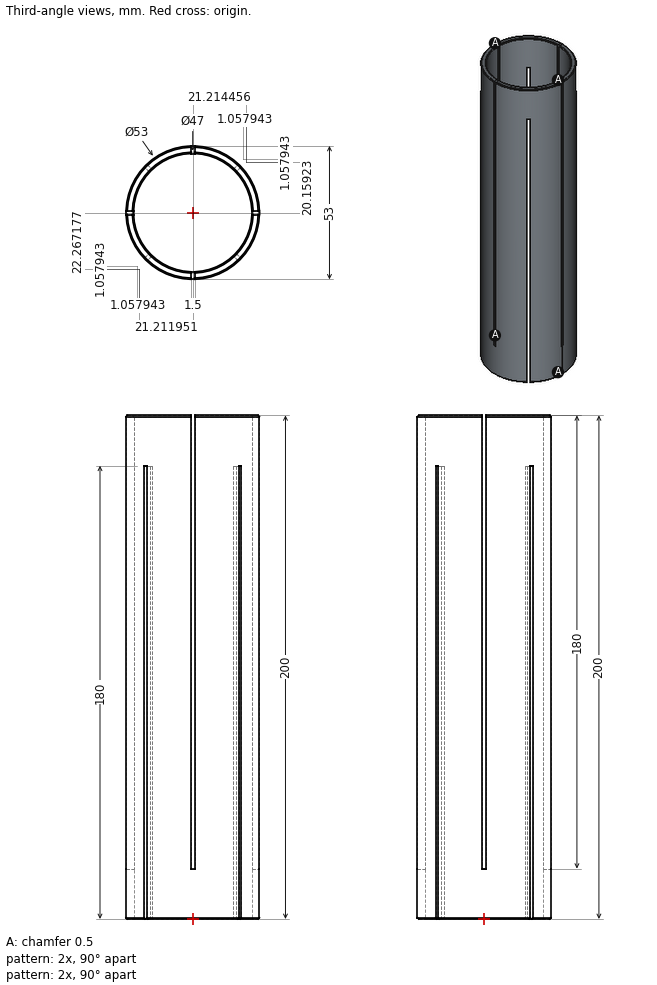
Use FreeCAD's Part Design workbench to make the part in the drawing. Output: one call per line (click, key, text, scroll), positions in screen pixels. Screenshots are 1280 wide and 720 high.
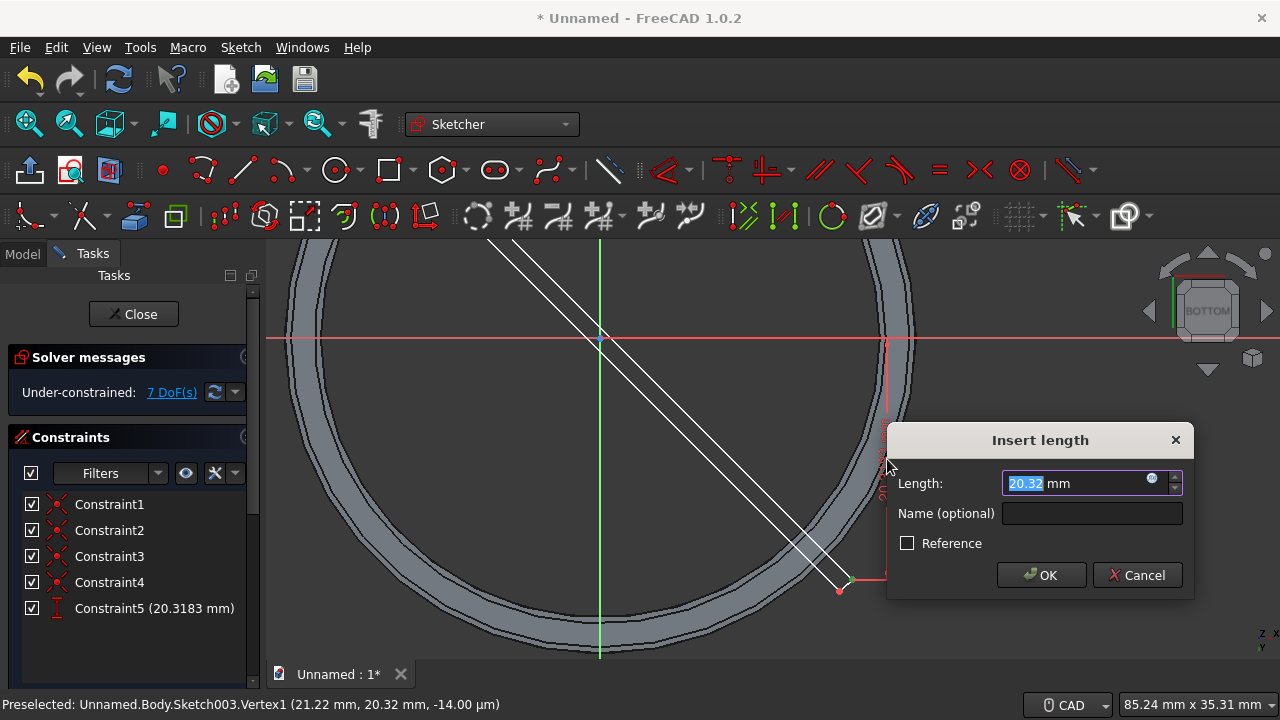
text(20.15923)
key(Return)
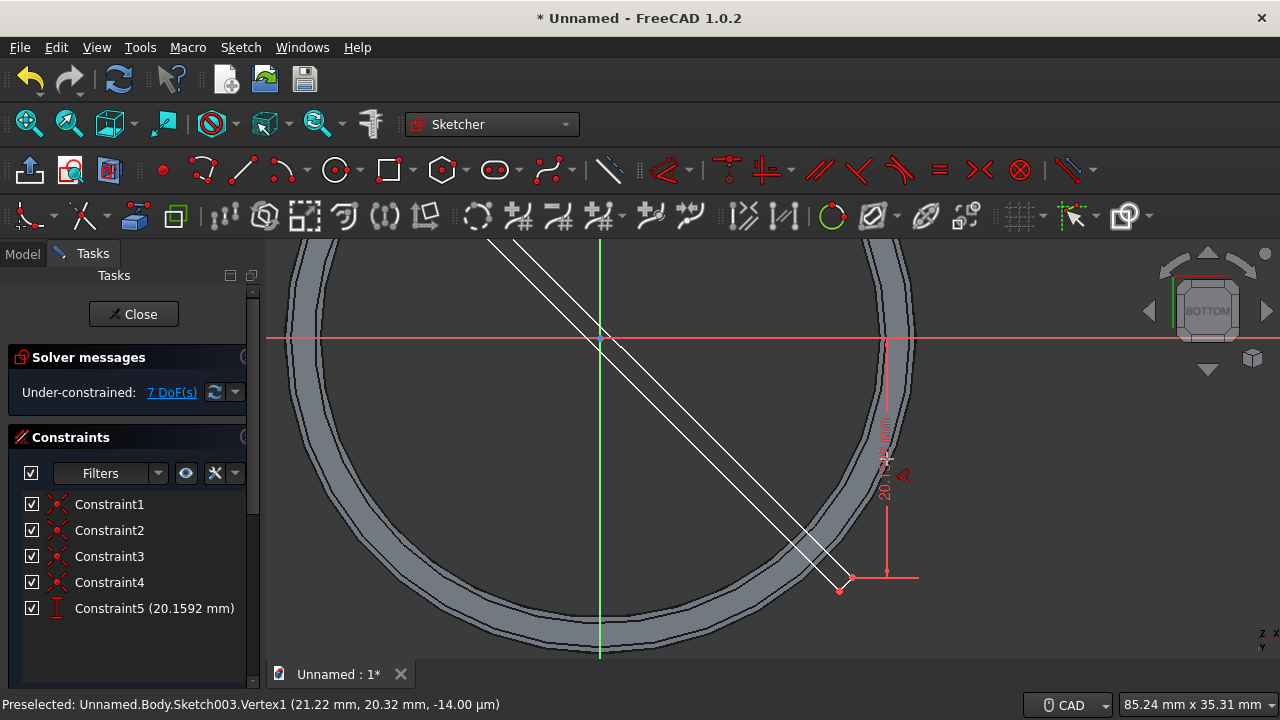
scroll(839, 592, down, 3)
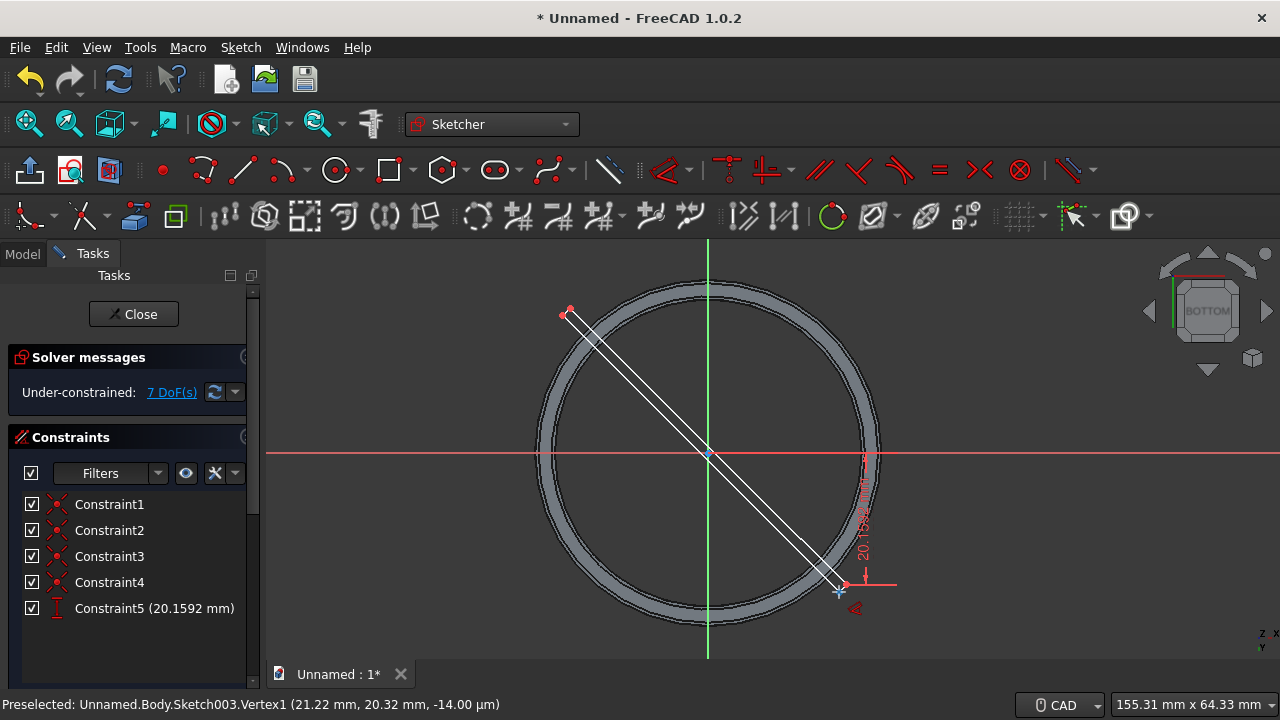
scroll(566, 312, up, 9)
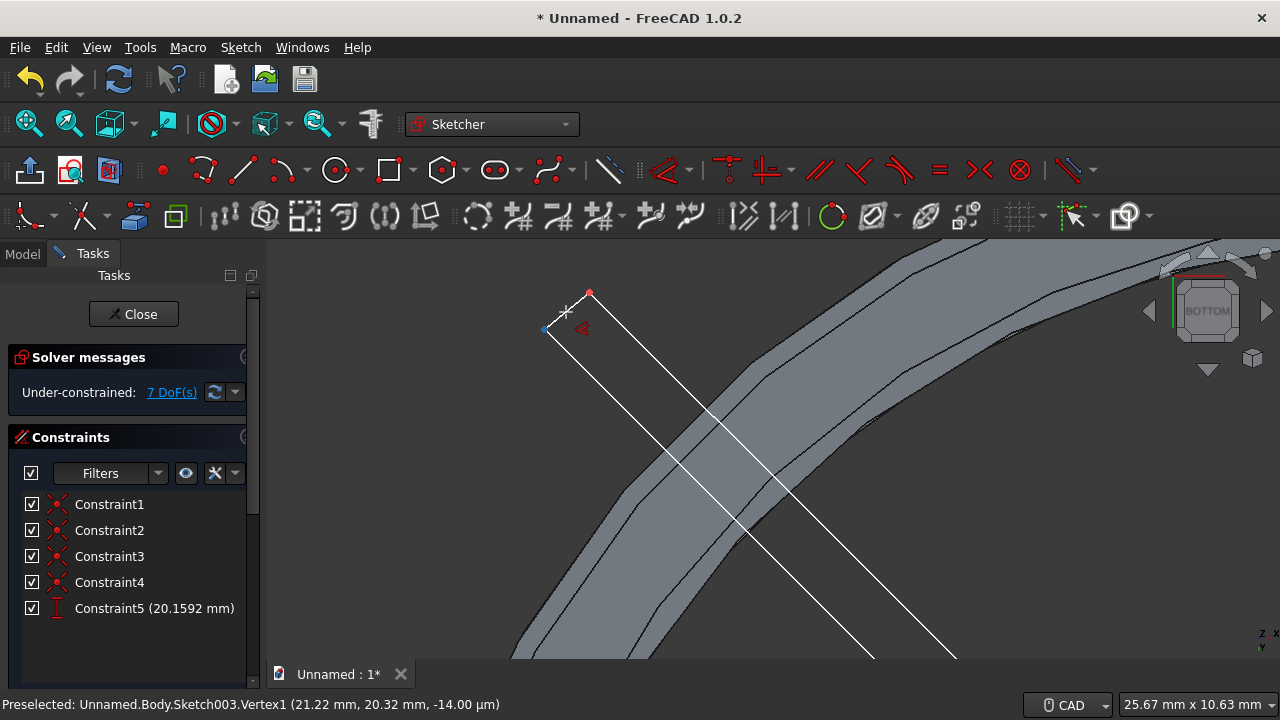
click(567, 311)
click(557, 363)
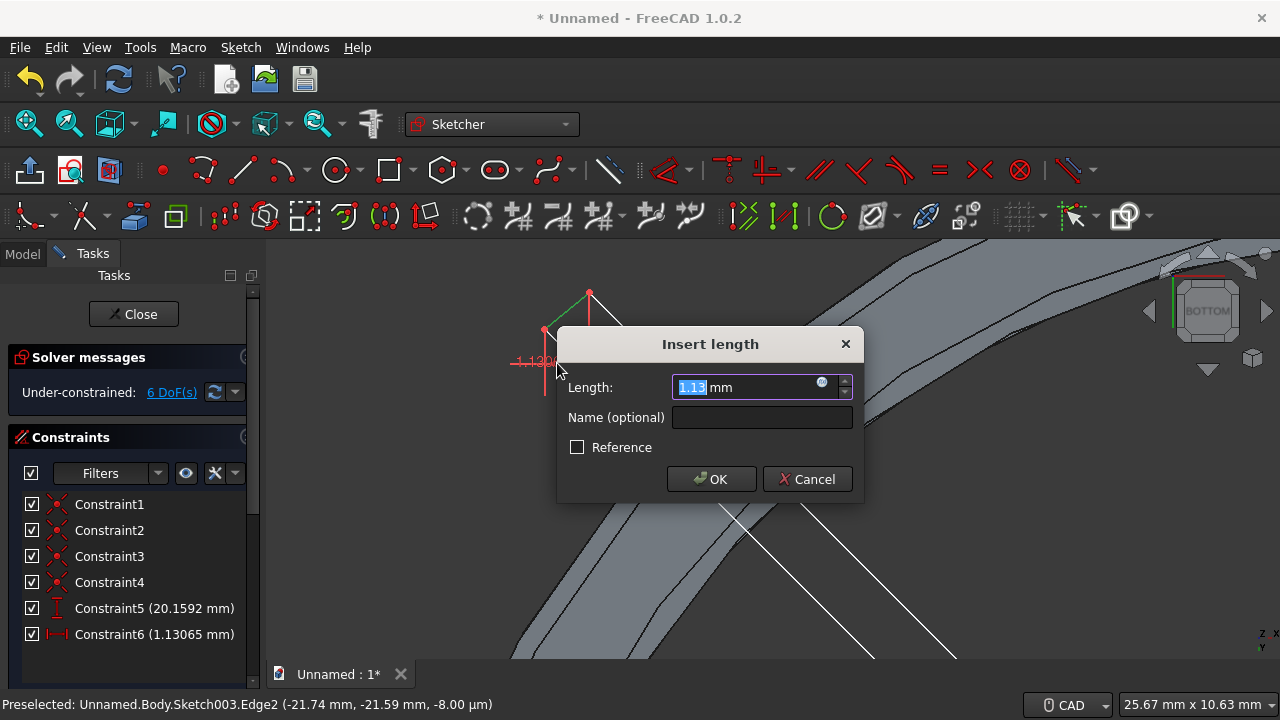
text(1.057943)
key(Return)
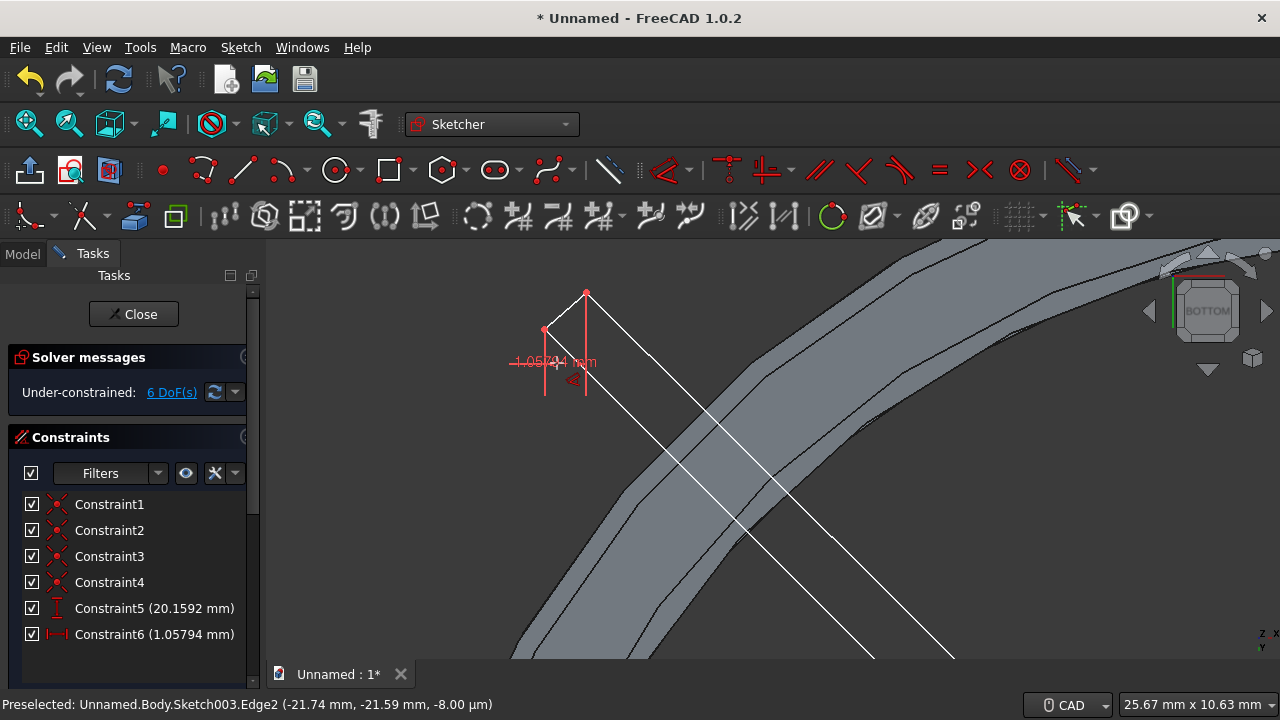
click(574, 304)
click(511, 311)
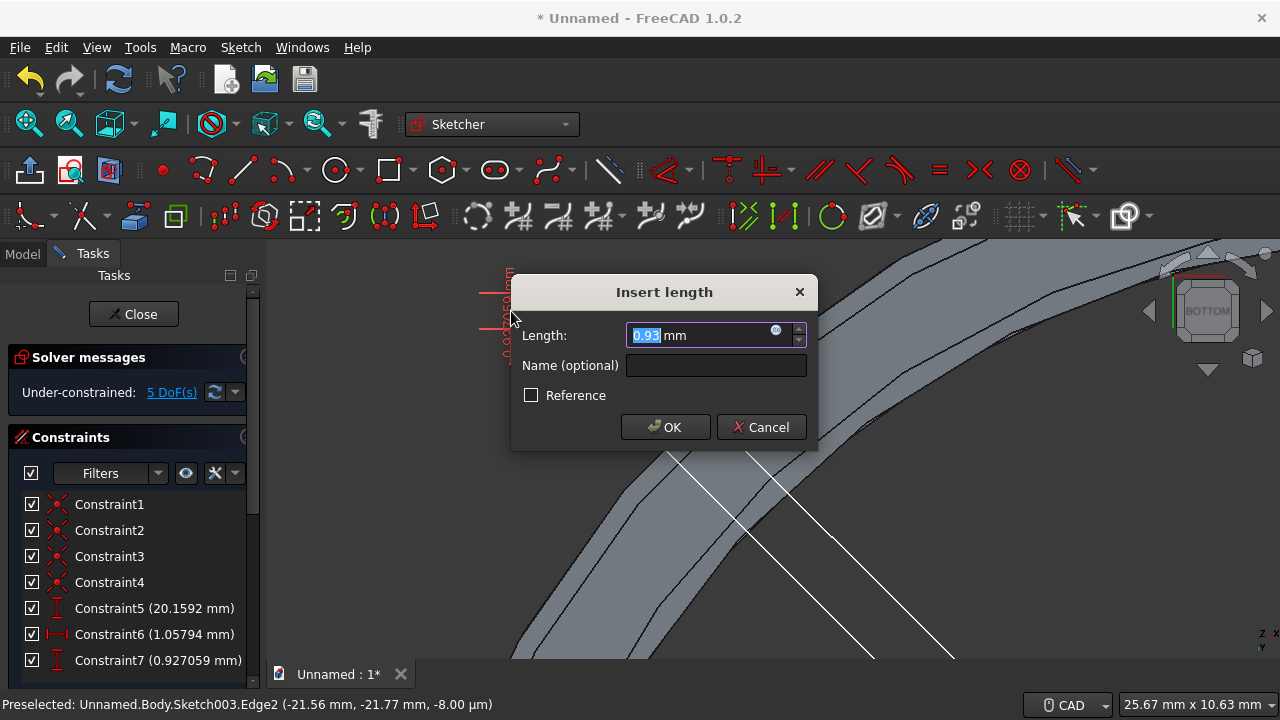
text(1.057943)
key(Return)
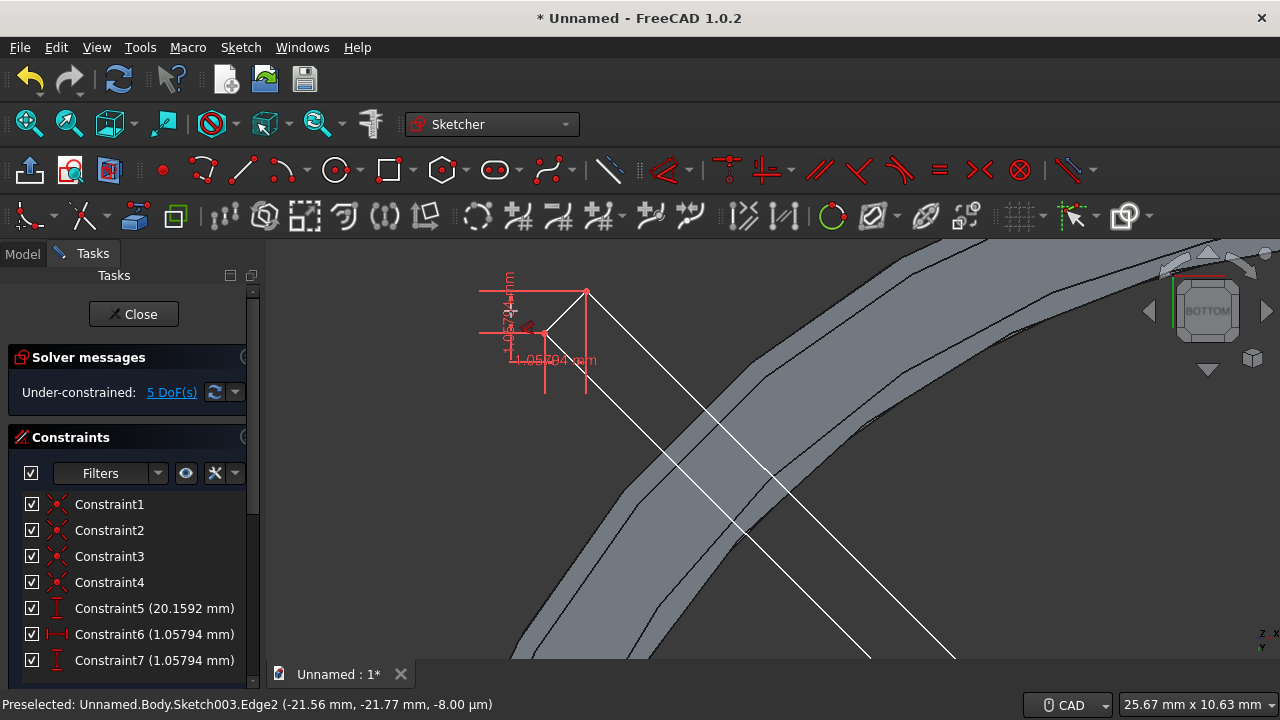
scroll(566, 311, down, 9)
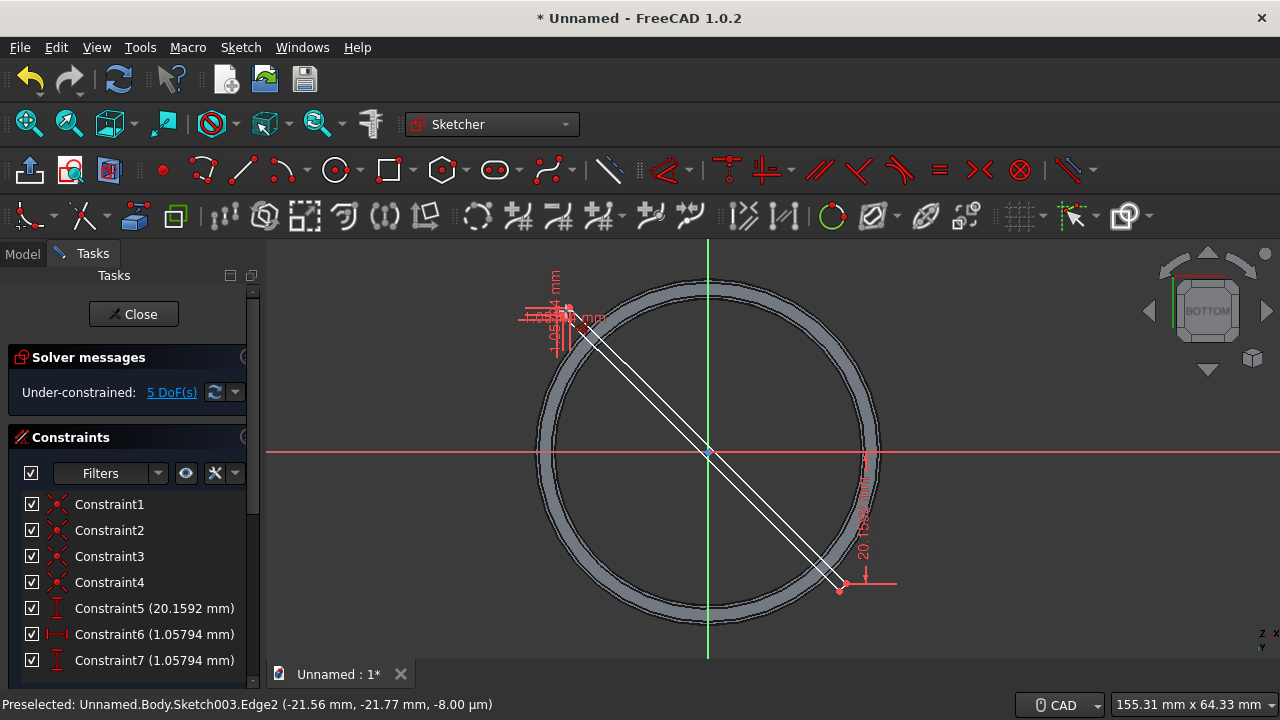
scroll(842, 589, up, 9)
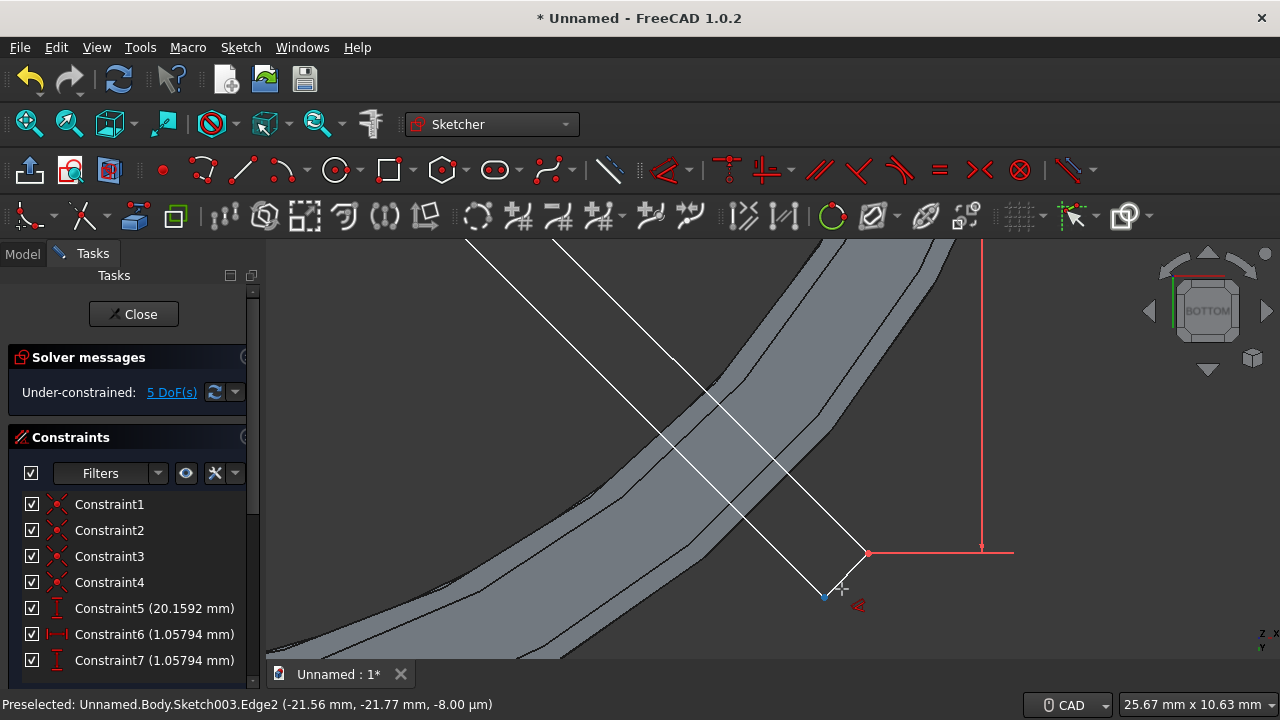
click(838, 585)
click(856, 519)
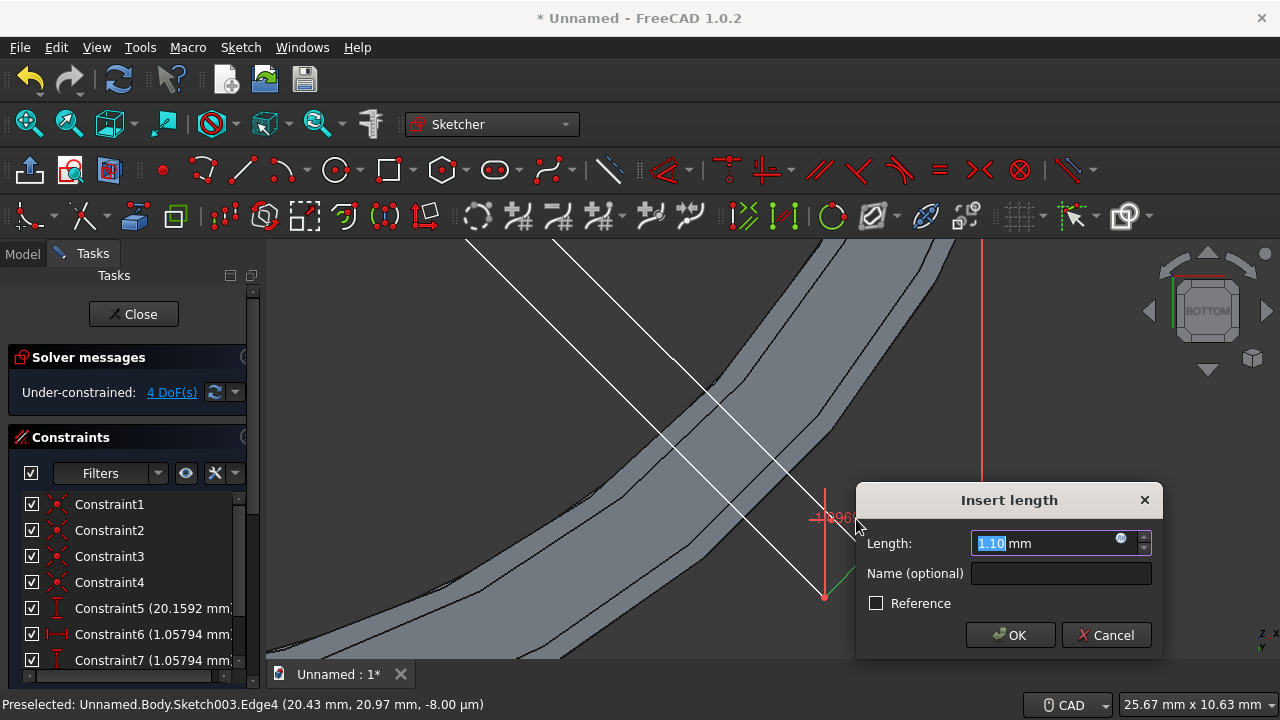
text(1.057943)
key(Return)